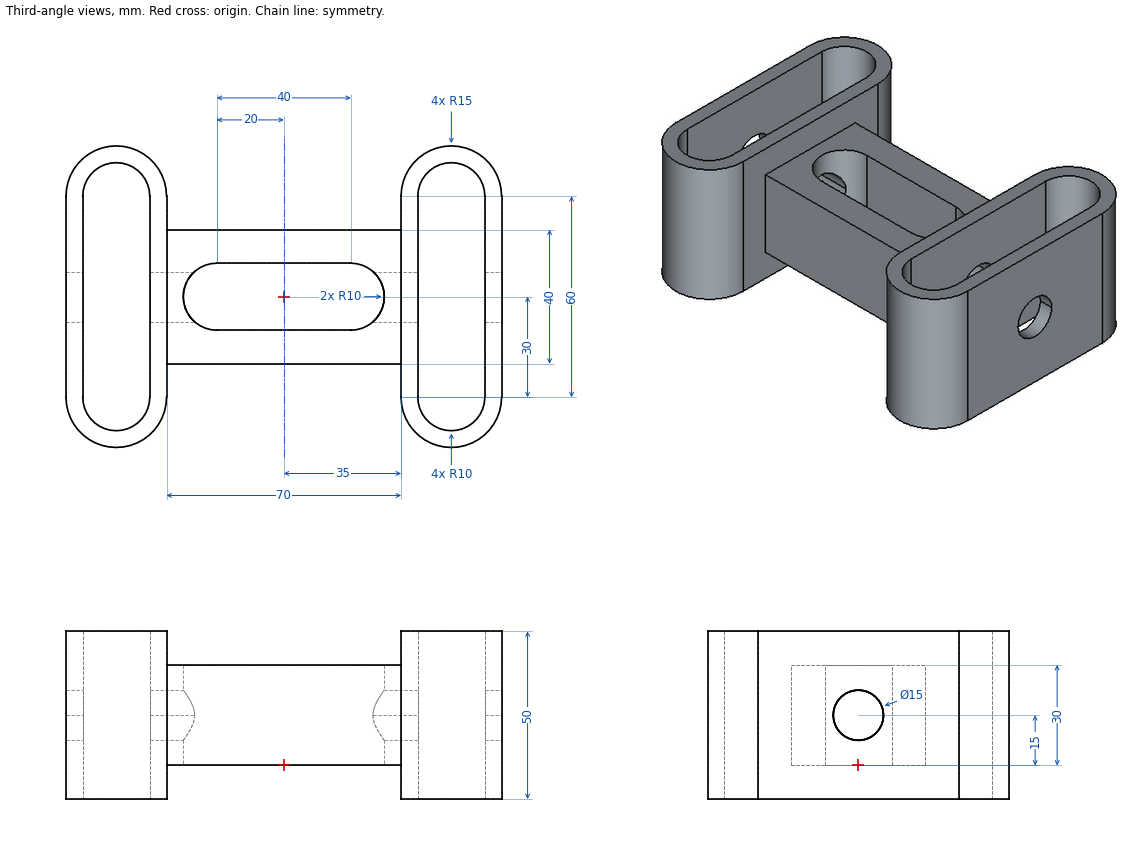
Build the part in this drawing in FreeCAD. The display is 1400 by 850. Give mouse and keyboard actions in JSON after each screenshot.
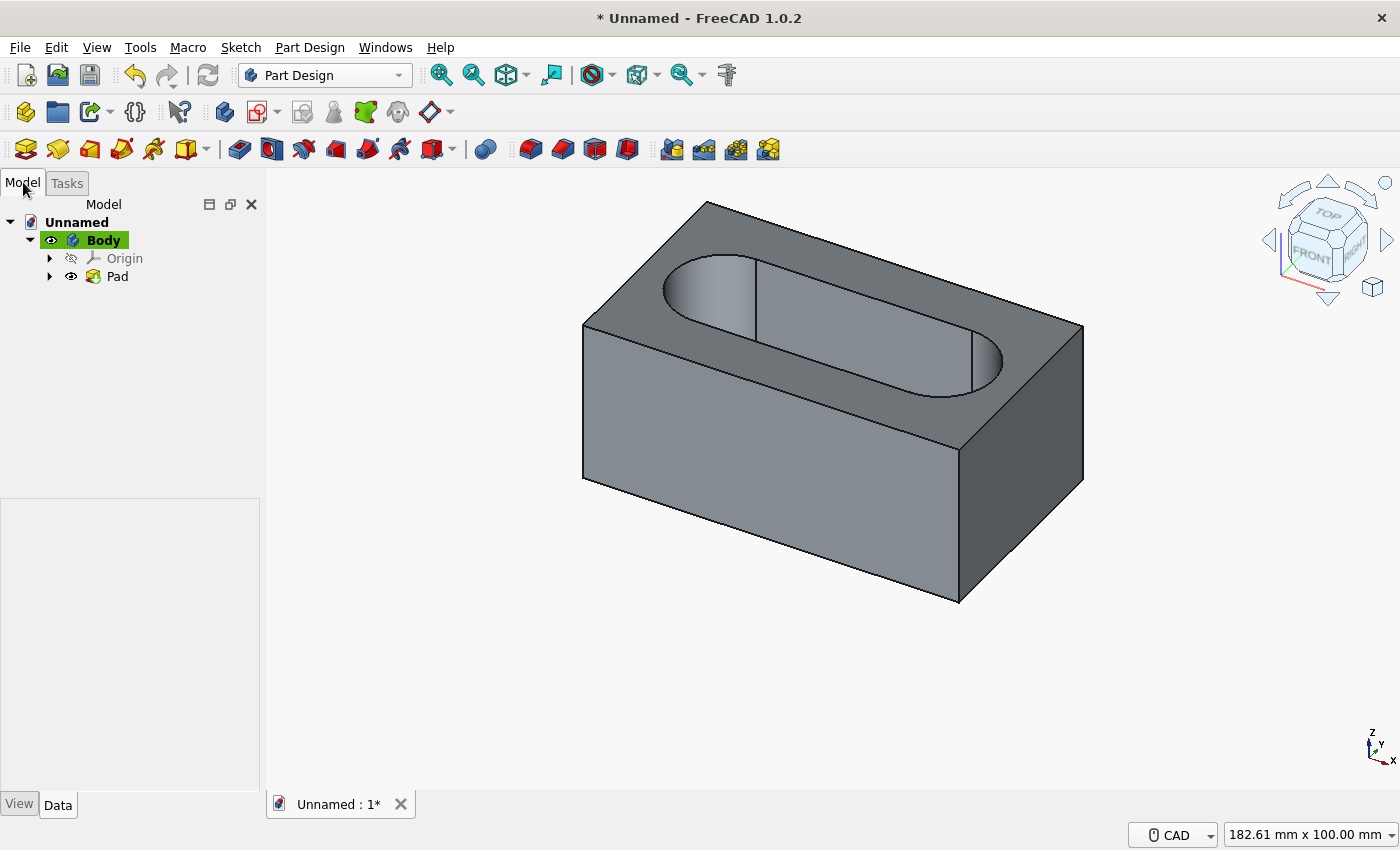
{"action": "left_click", "coordinate": [50, 258]}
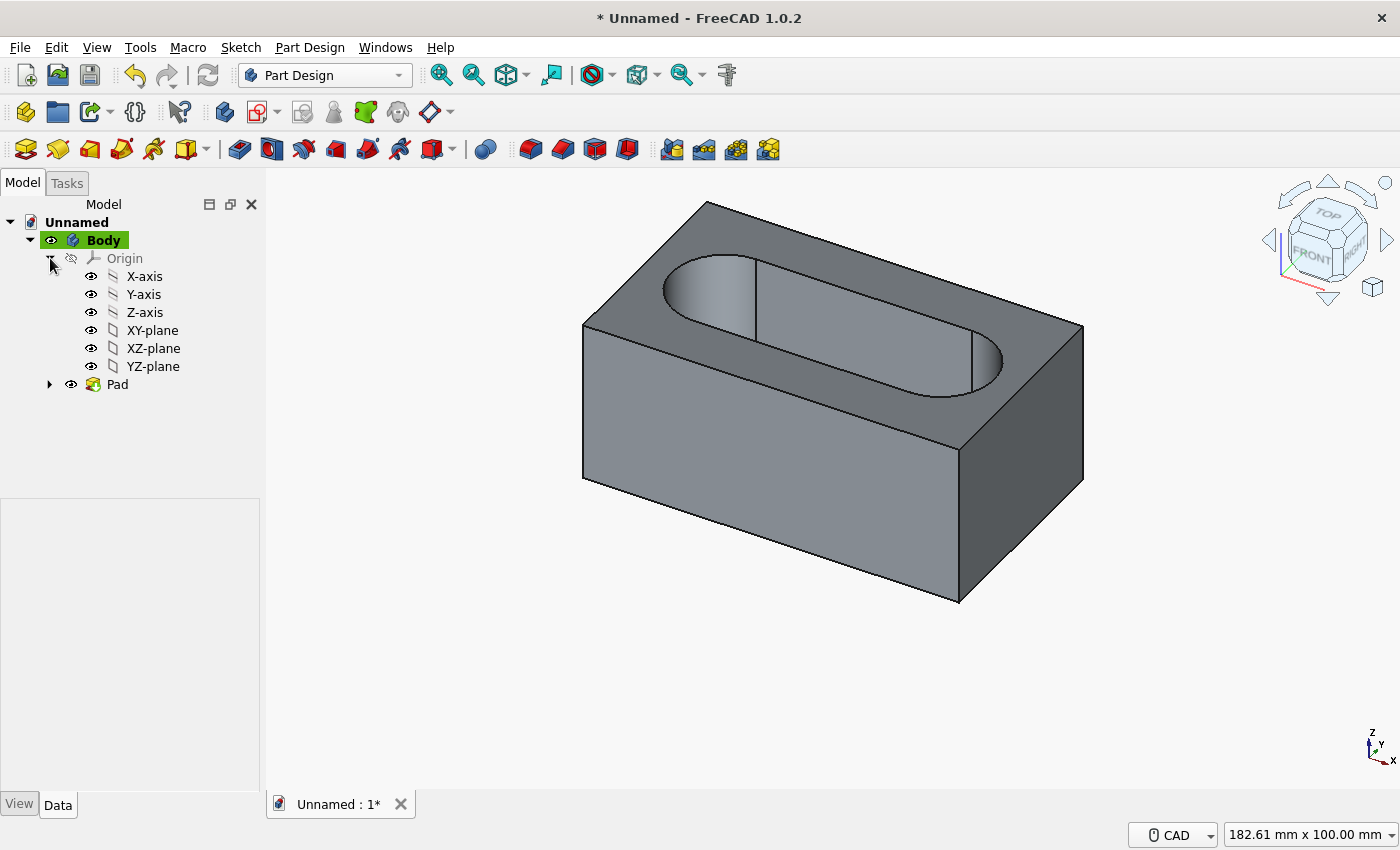
{"action": "left_click", "coordinate": [136, 330]}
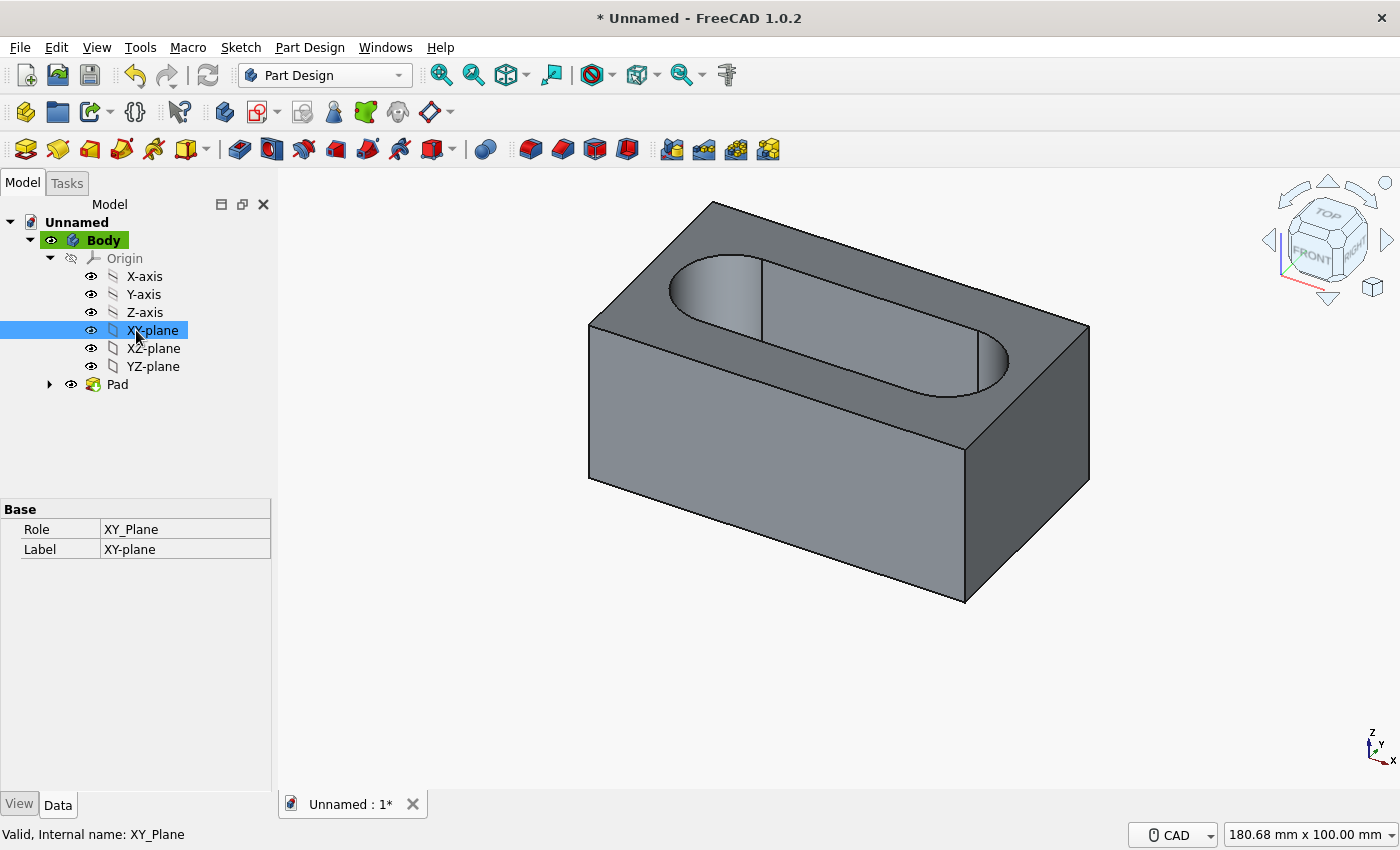
{"action": "left_click", "coordinate": [430, 112]}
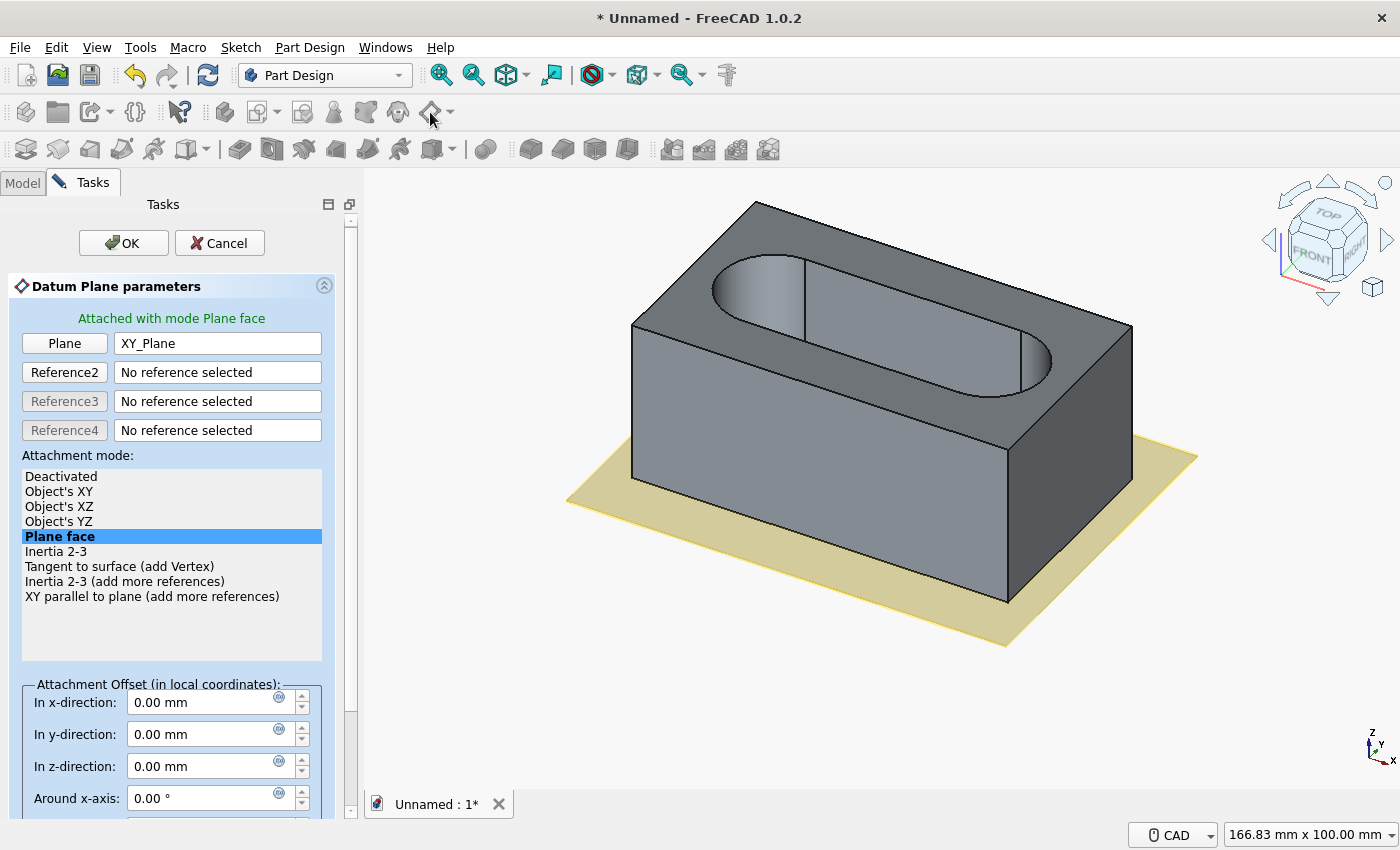
{"action": "triple_click", "coordinate": [210, 766]}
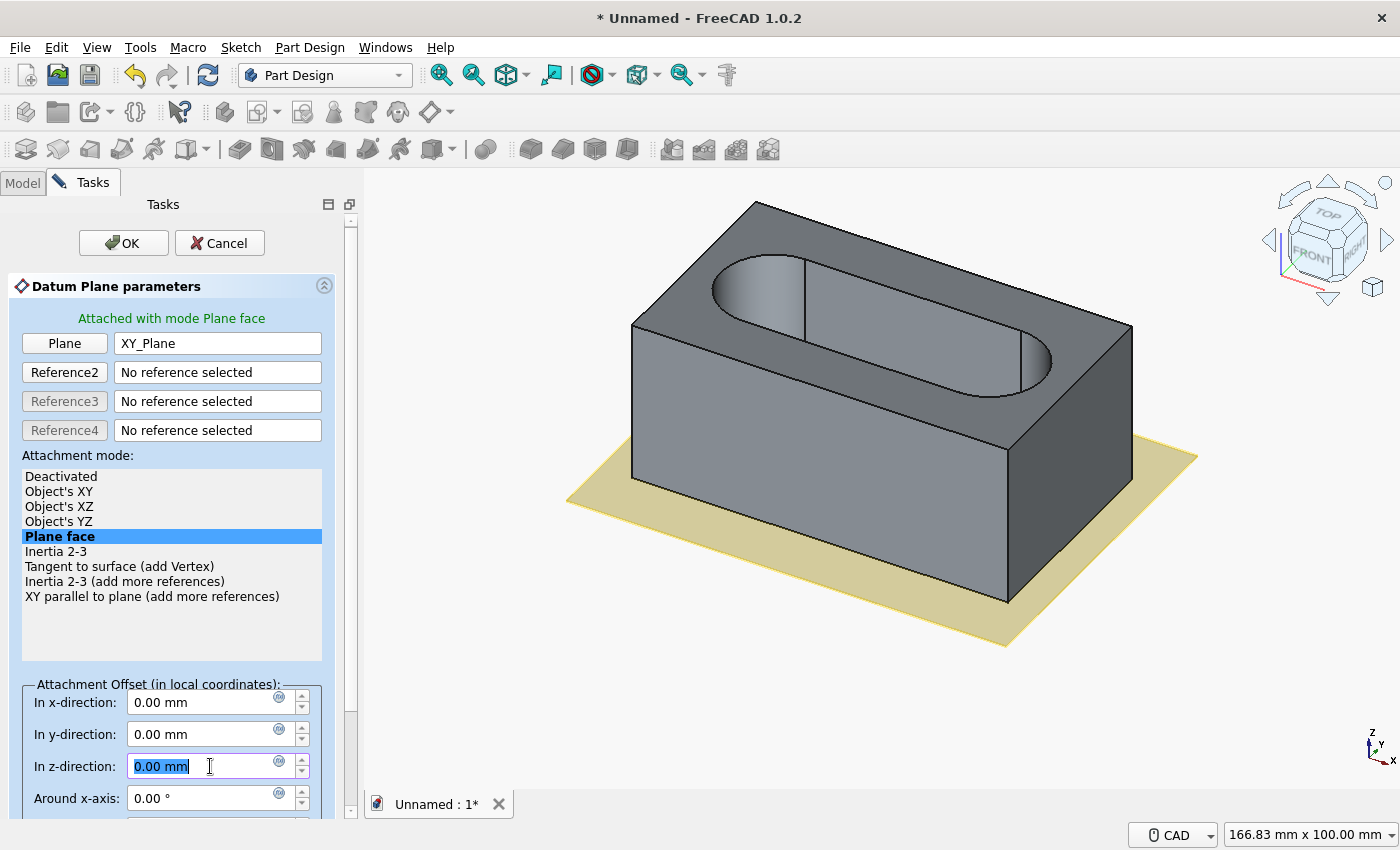
{"action": "type", "text": "15"}
{"action": "key", "text": "Tab"}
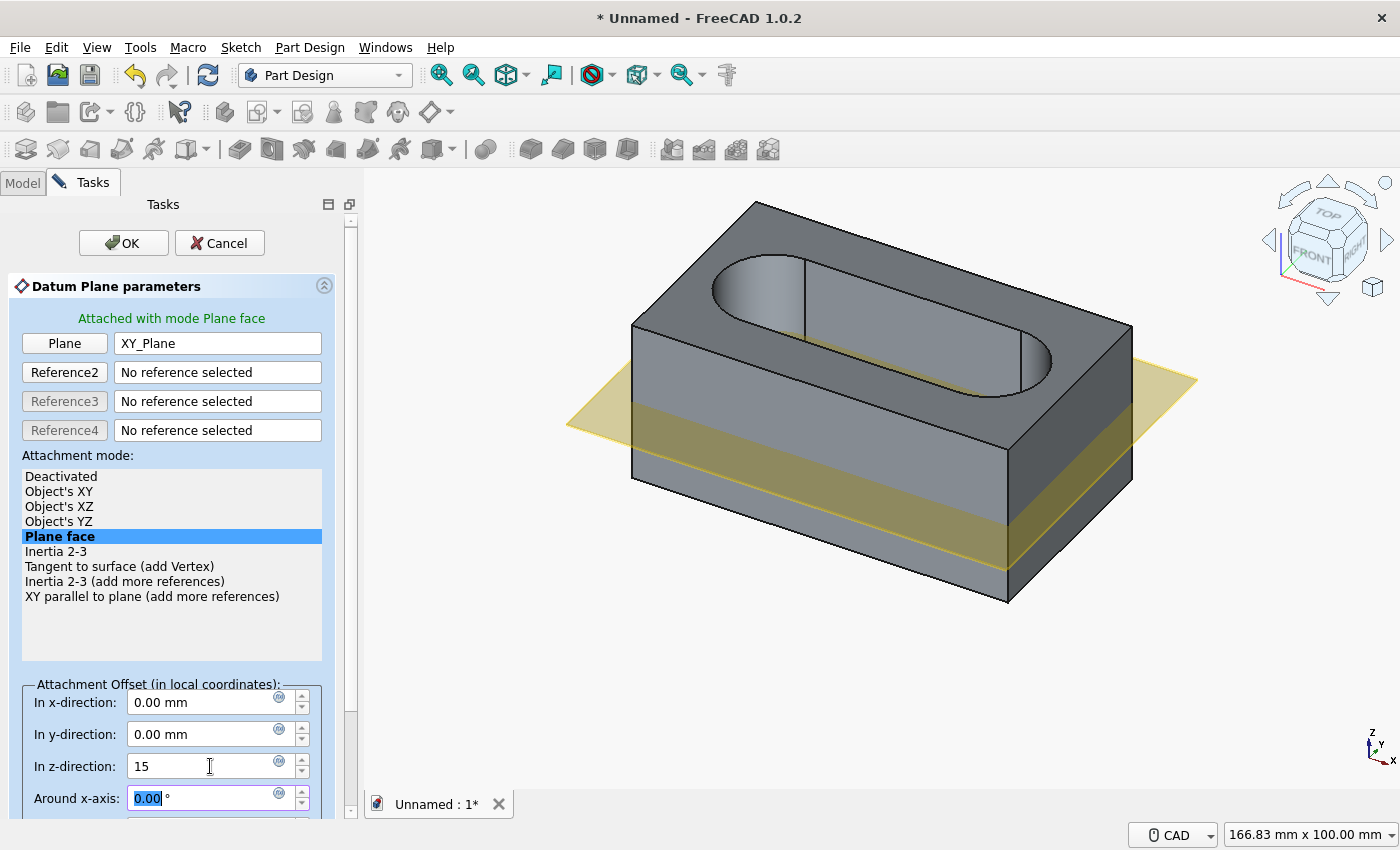
{"action": "left_click", "coordinate": [124, 243]}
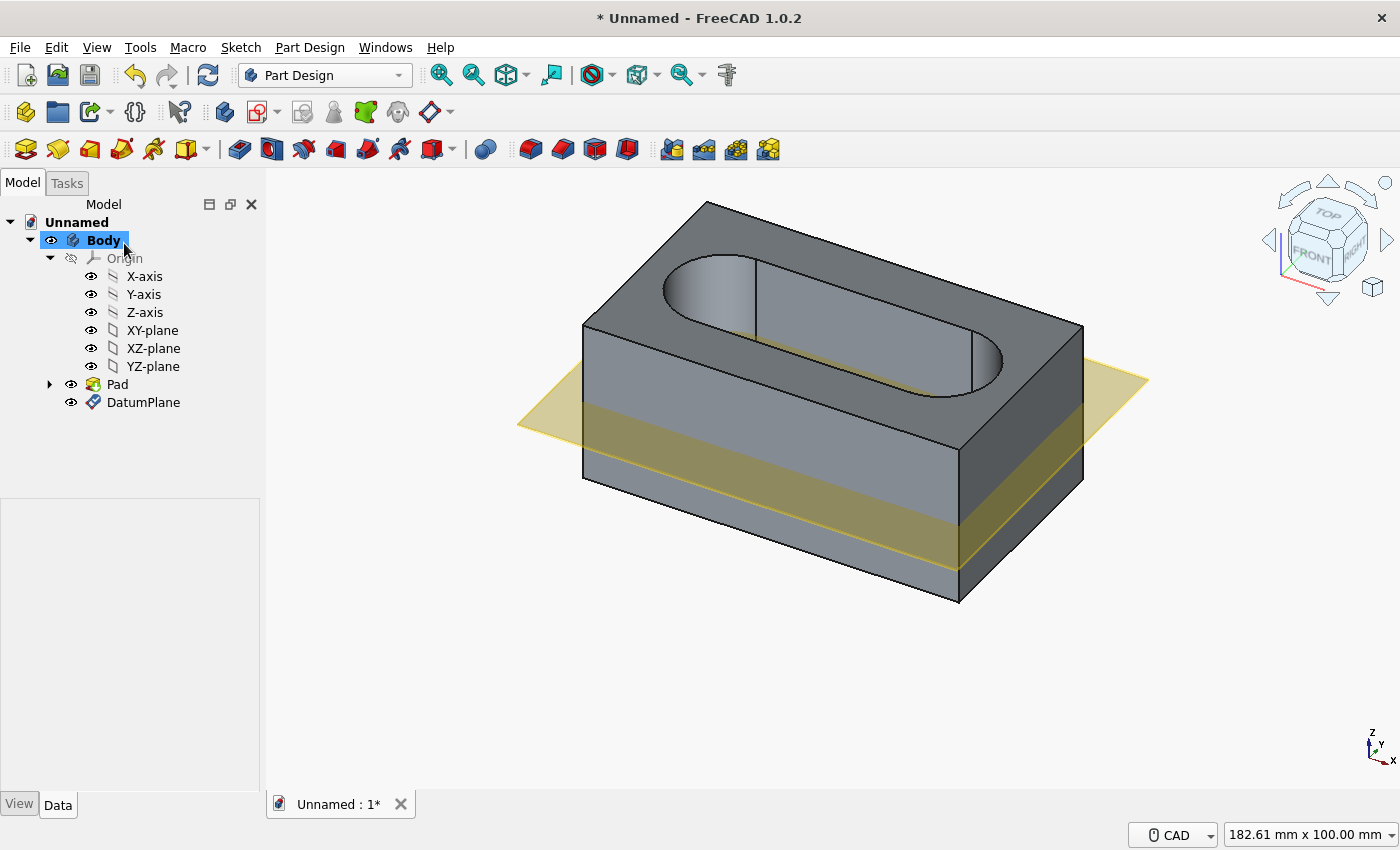
{"action": "left_click", "coordinate": [116, 402]}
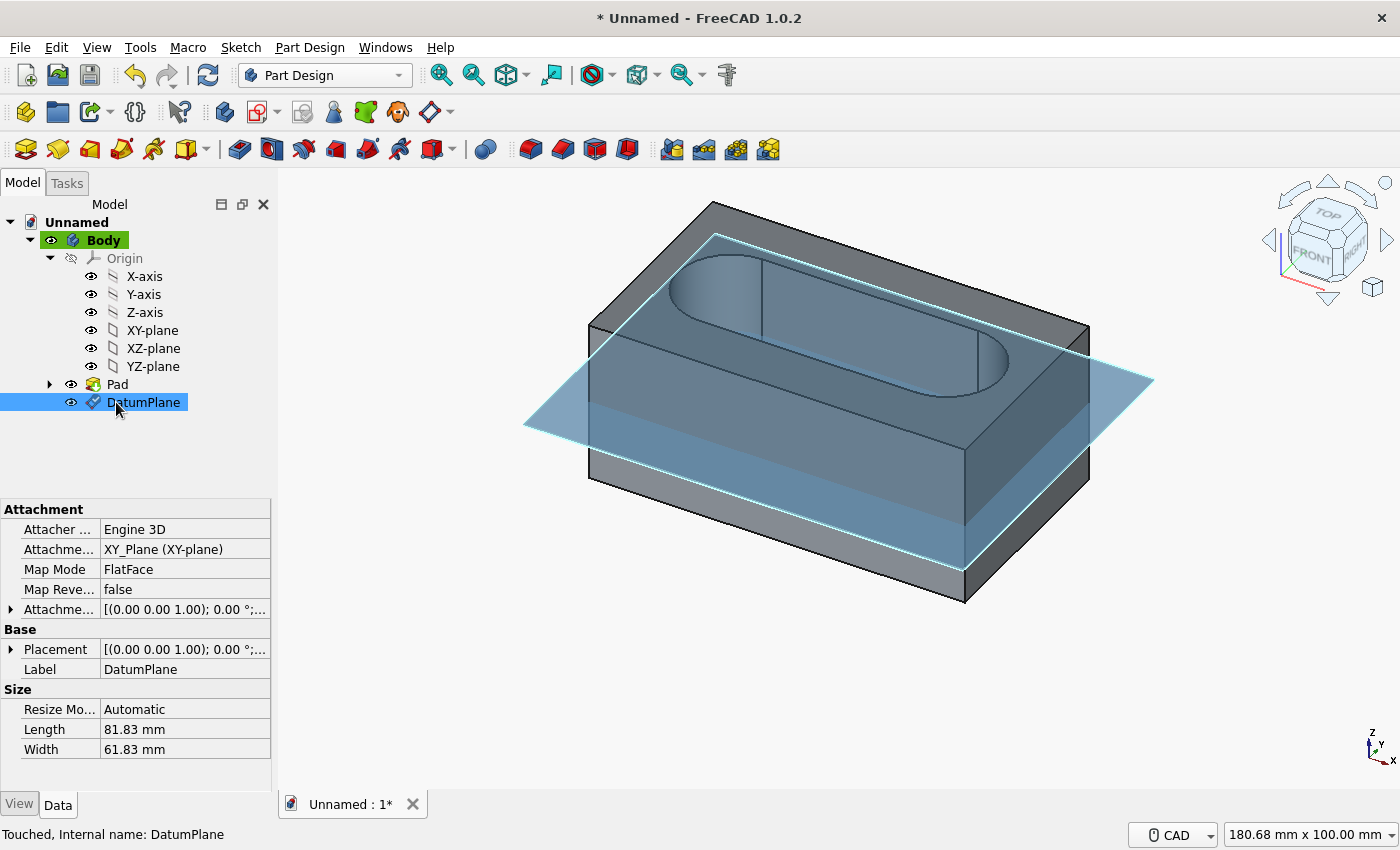
{"action": "left_click", "coordinate": [258, 112]}